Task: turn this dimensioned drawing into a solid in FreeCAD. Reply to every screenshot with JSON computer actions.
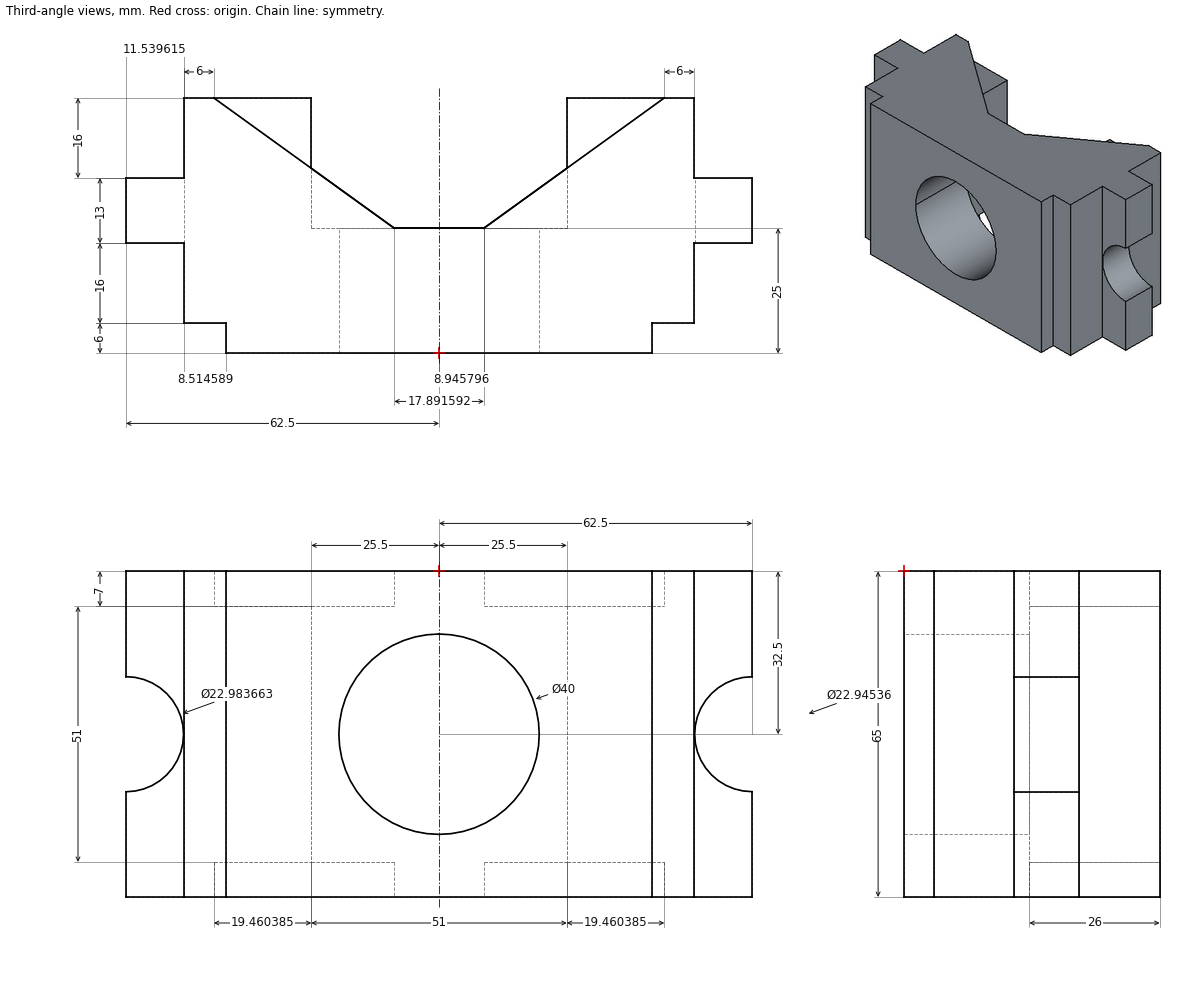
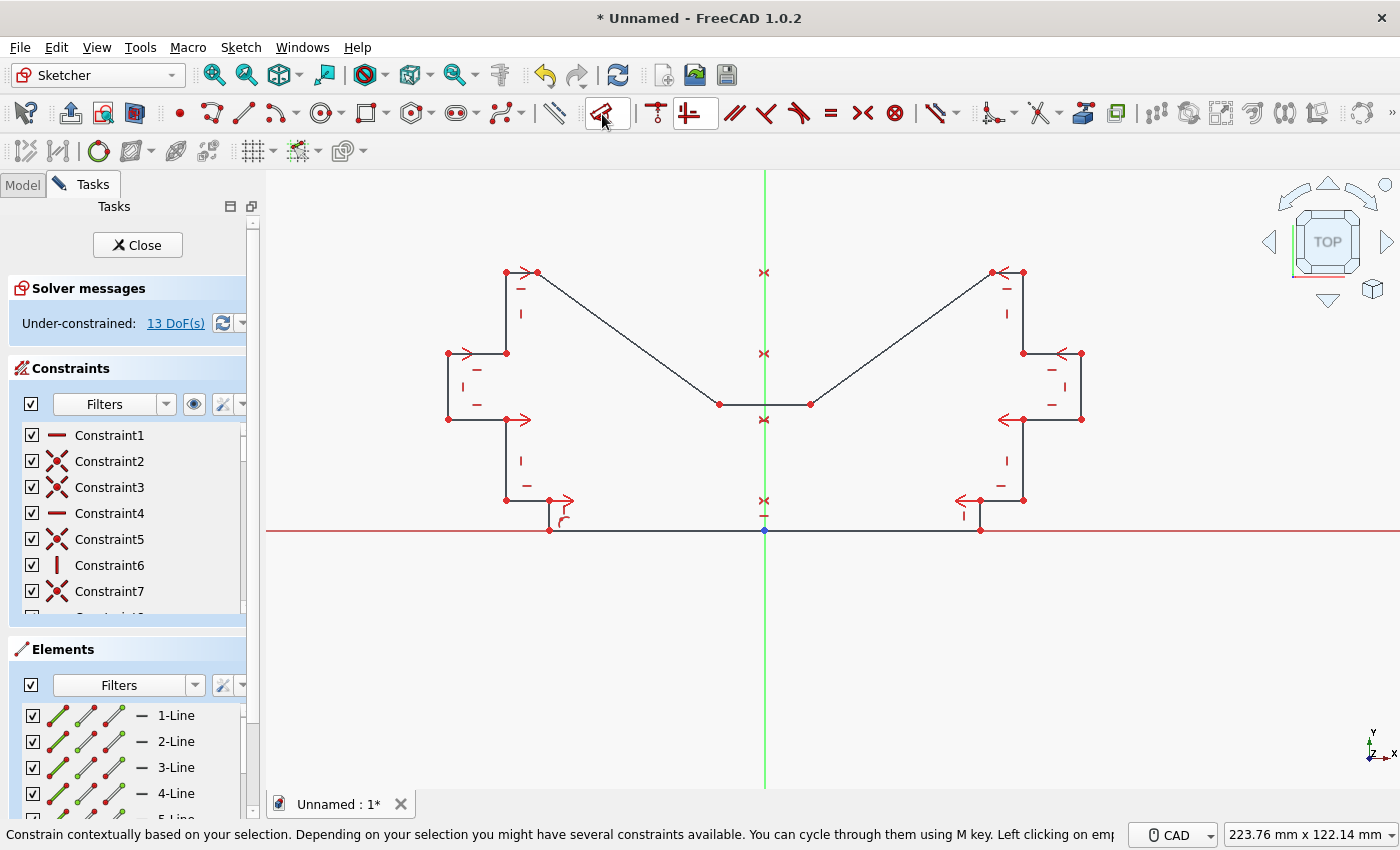
{"action": "scroll", "coordinate": [528, 273], "scroll_direction": "up", "scroll_amount": 2}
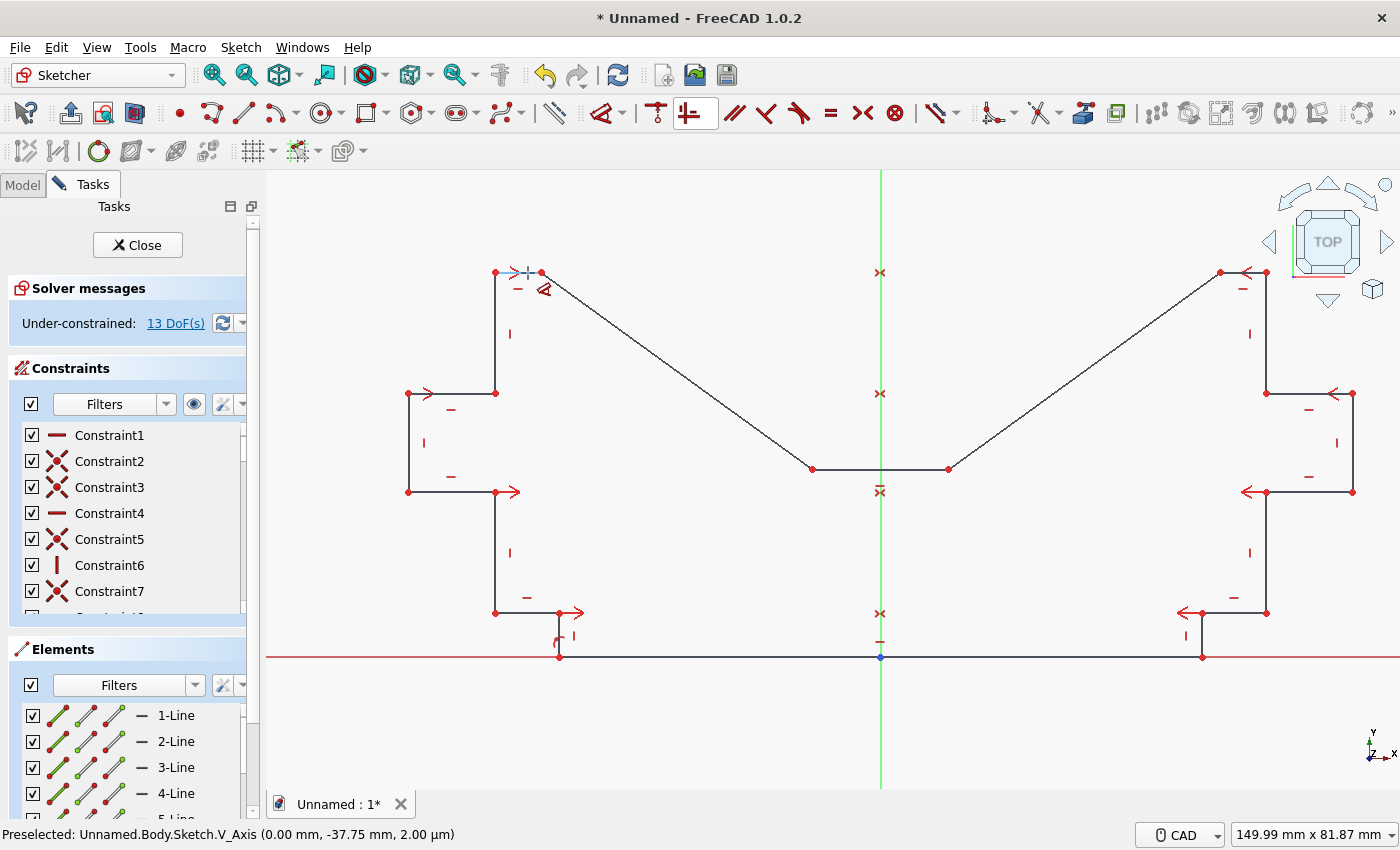
{"action": "left_click", "coordinate": [527, 273]}
{"action": "left_click", "coordinate": [518, 239]}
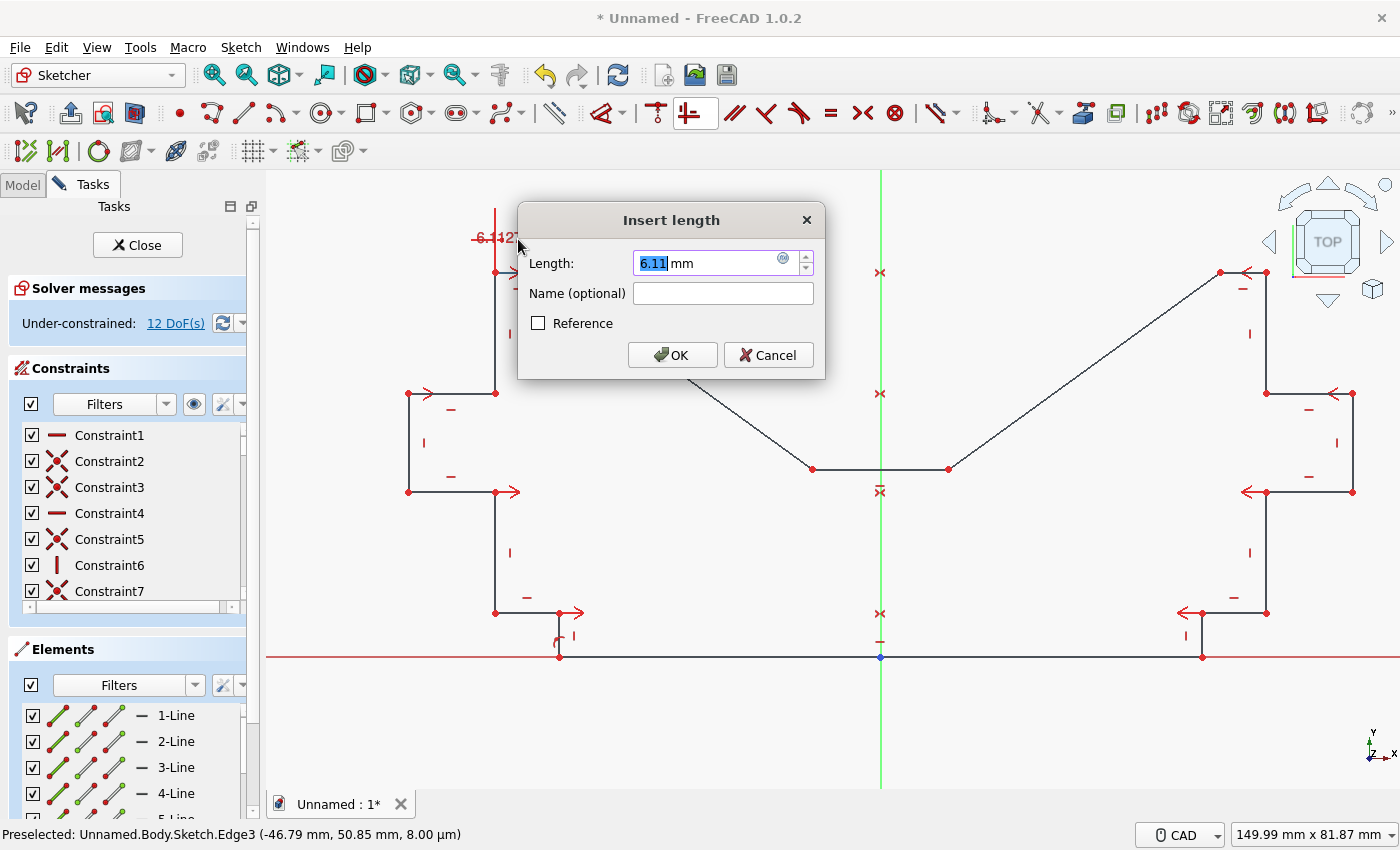
{"action": "type", "text": "6"}
{"action": "key", "text": "Return"}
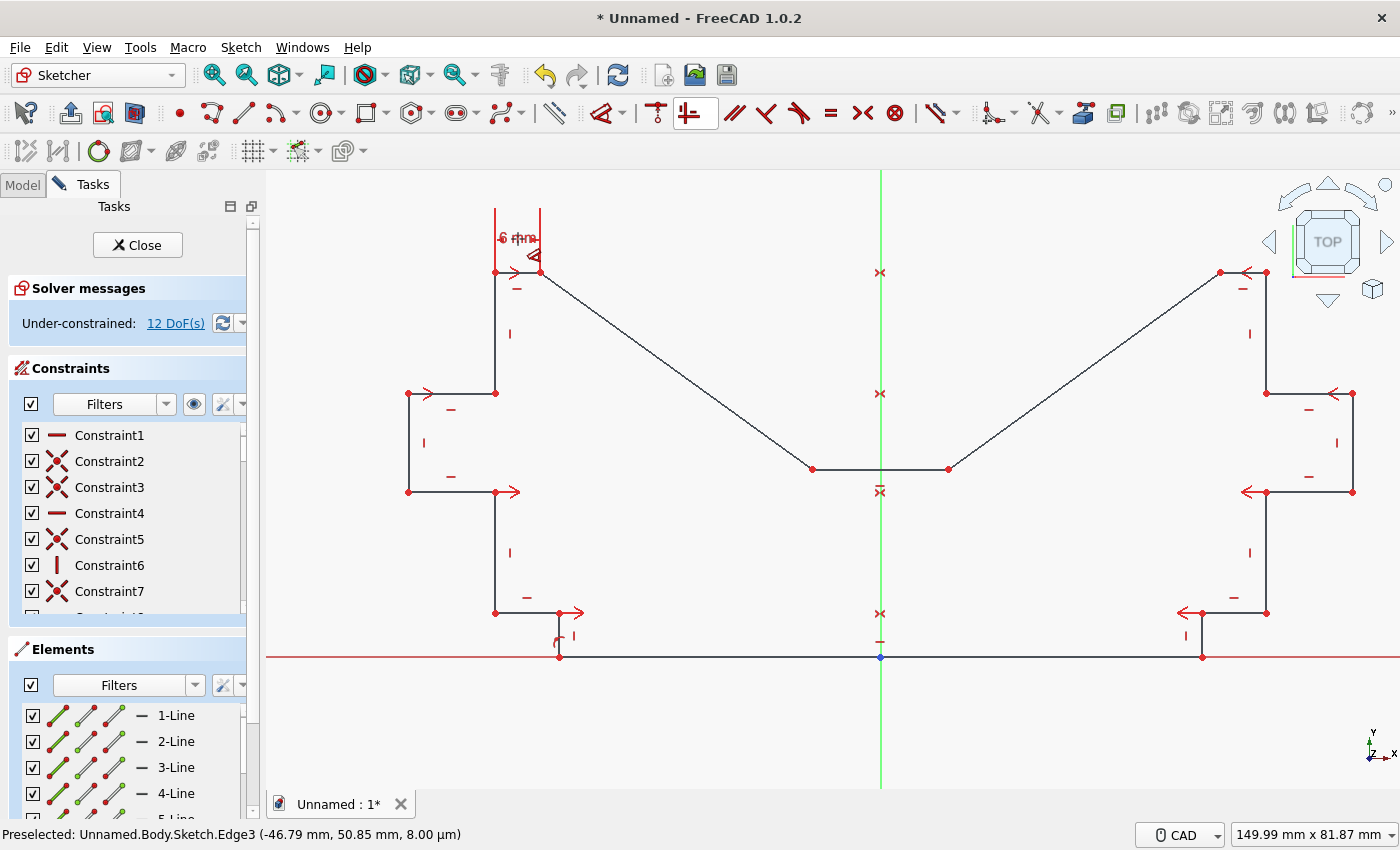
{"action": "left_click", "coordinate": [559, 626]}
{"action": "left_click", "coordinate": [525, 635]}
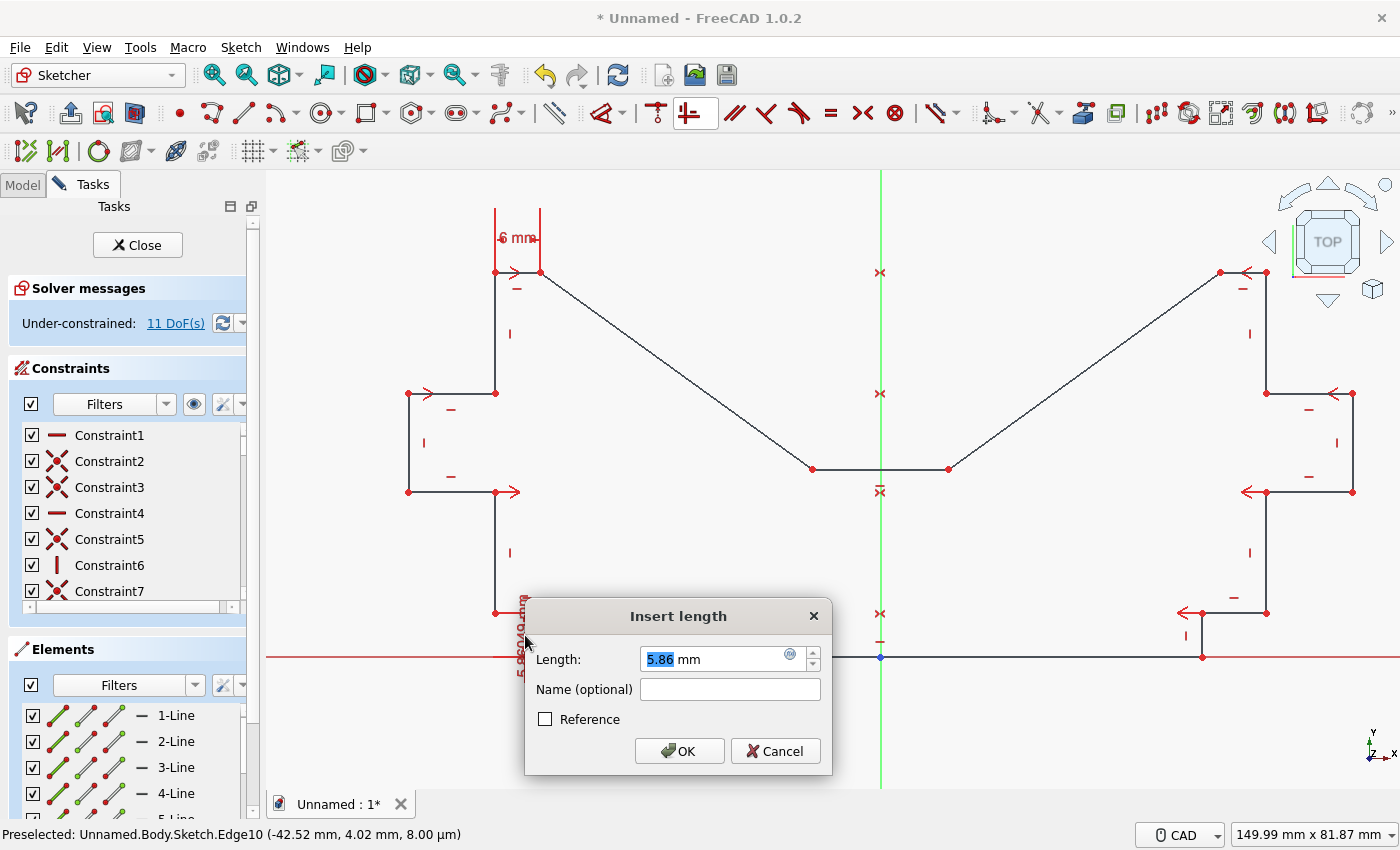
{"action": "type", "text": "6"}
{"action": "key", "text": "Return"}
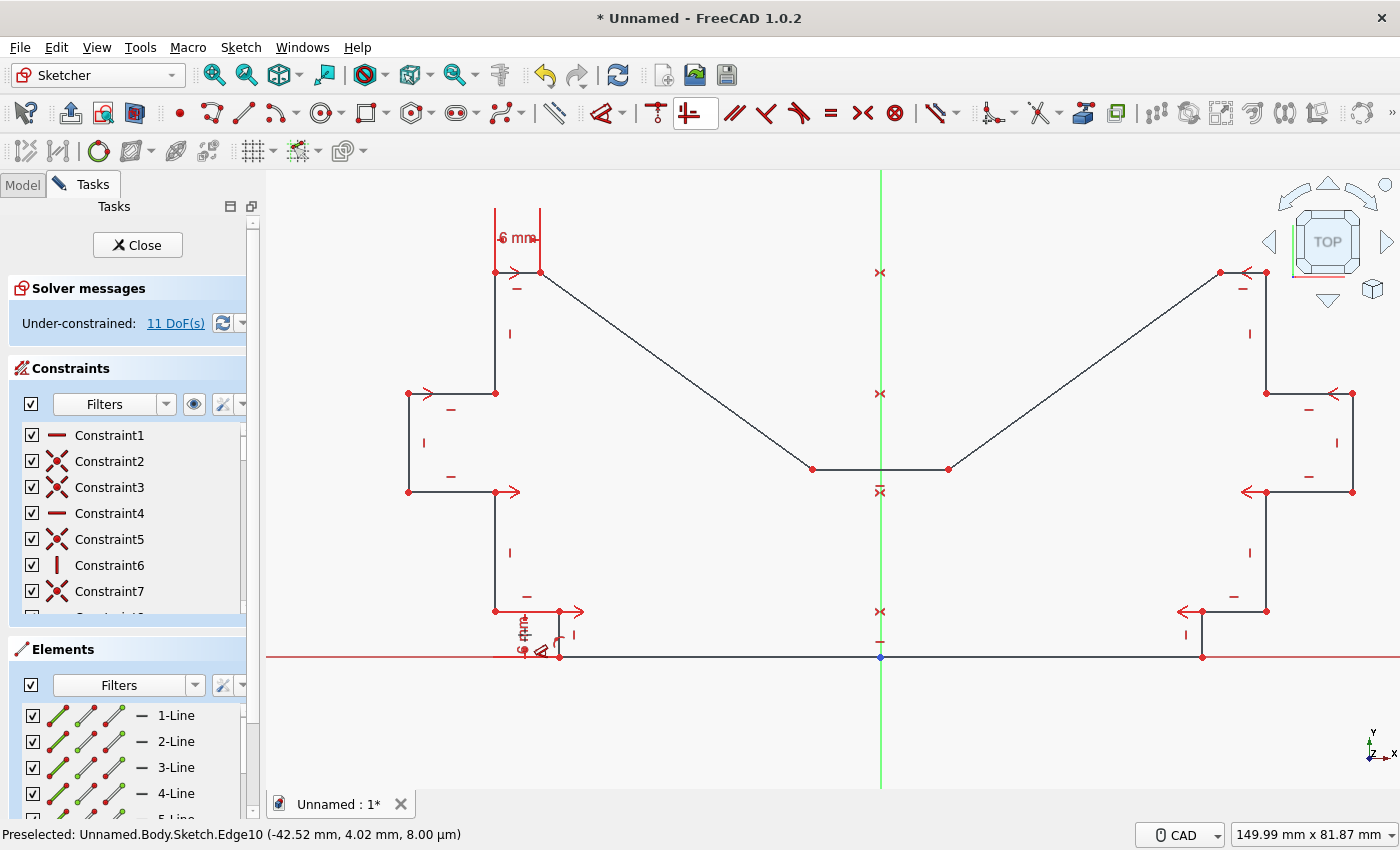
{"action": "left_click", "coordinate": [1234, 273]}
{"action": "left_click", "coordinate": [1228, 239]}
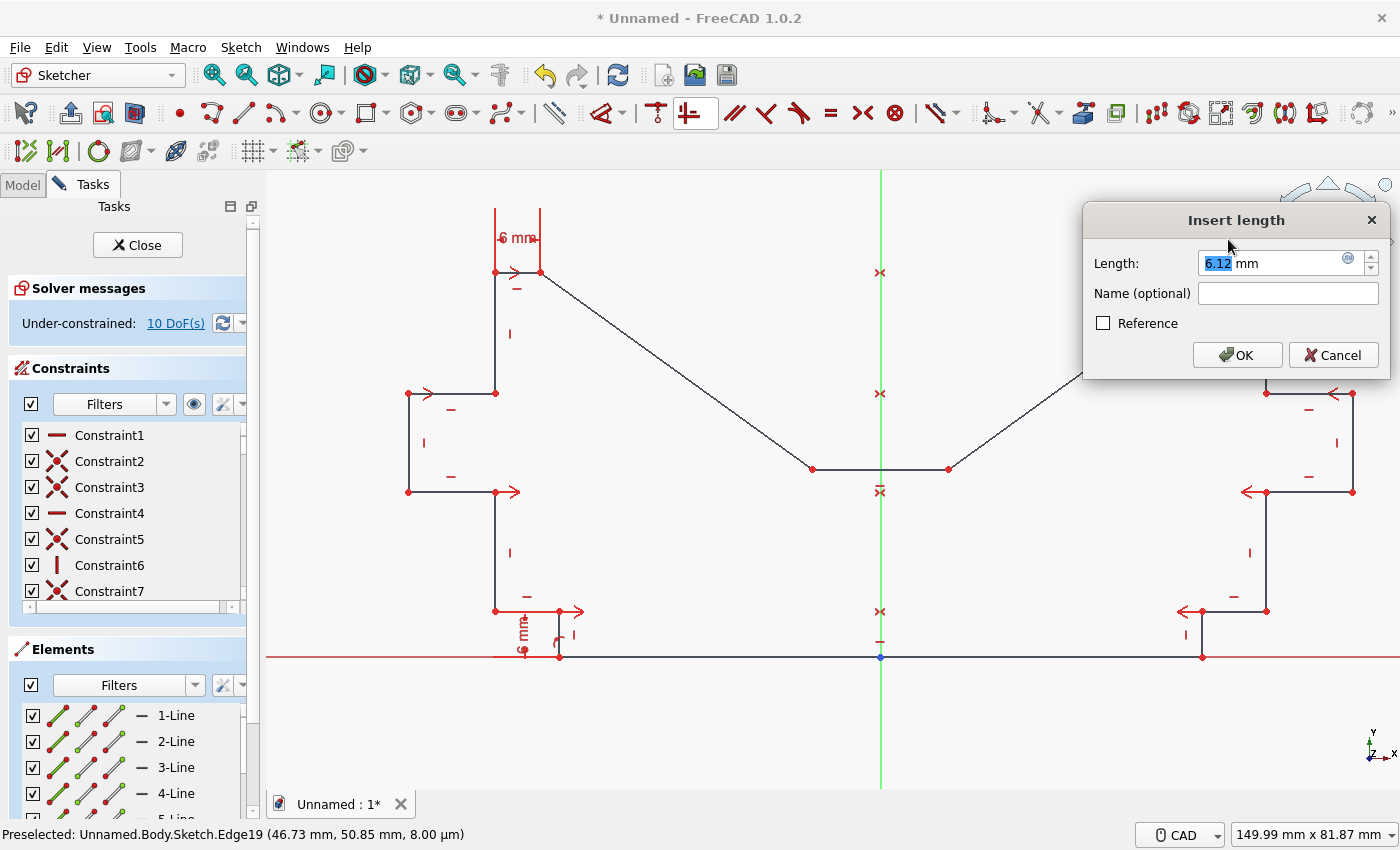
{"action": "type", "text": "6"}
{"action": "key", "text": "Return"}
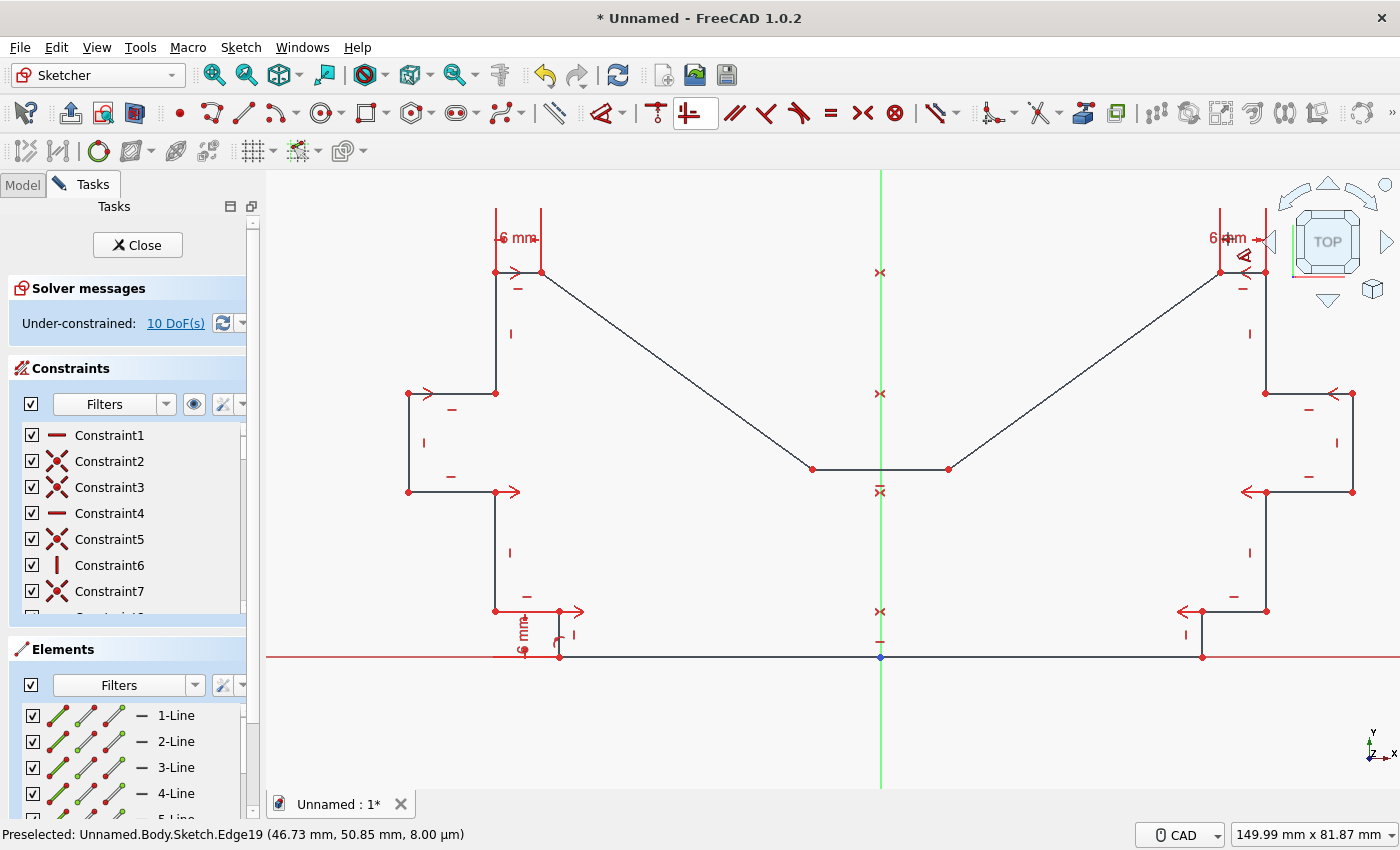
{"action": "left_click", "coordinate": [496, 309]}
{"action": "left_click", "coordinate": [462, 333]}